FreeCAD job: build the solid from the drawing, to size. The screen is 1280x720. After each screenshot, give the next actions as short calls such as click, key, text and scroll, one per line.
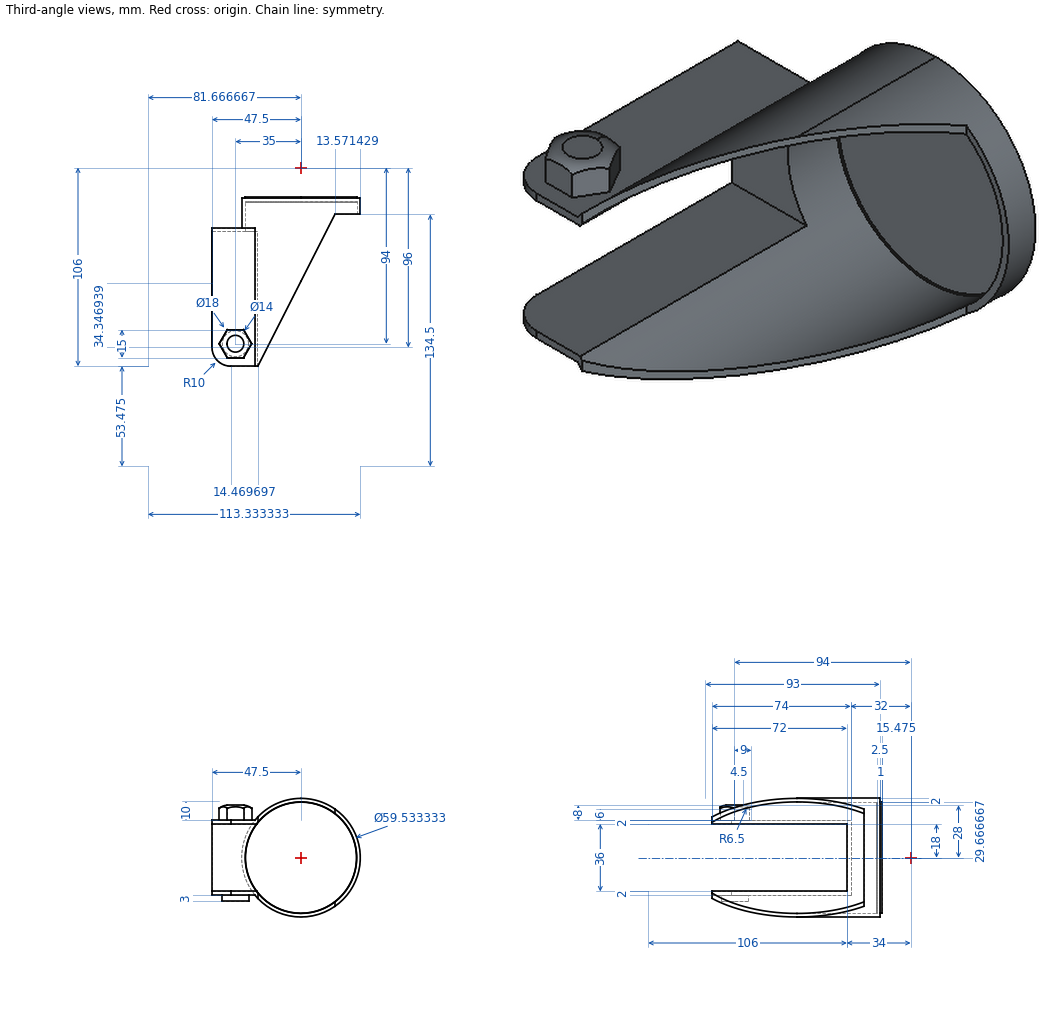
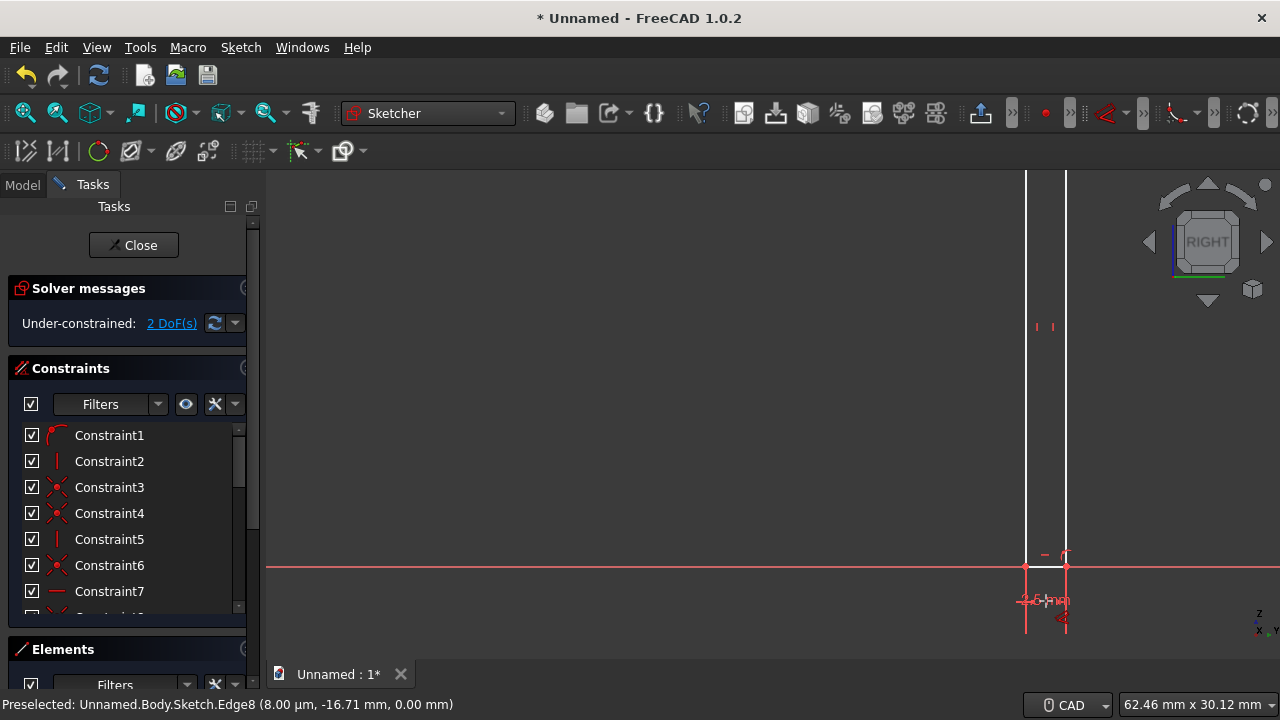
scroll(823, 460, down, 6)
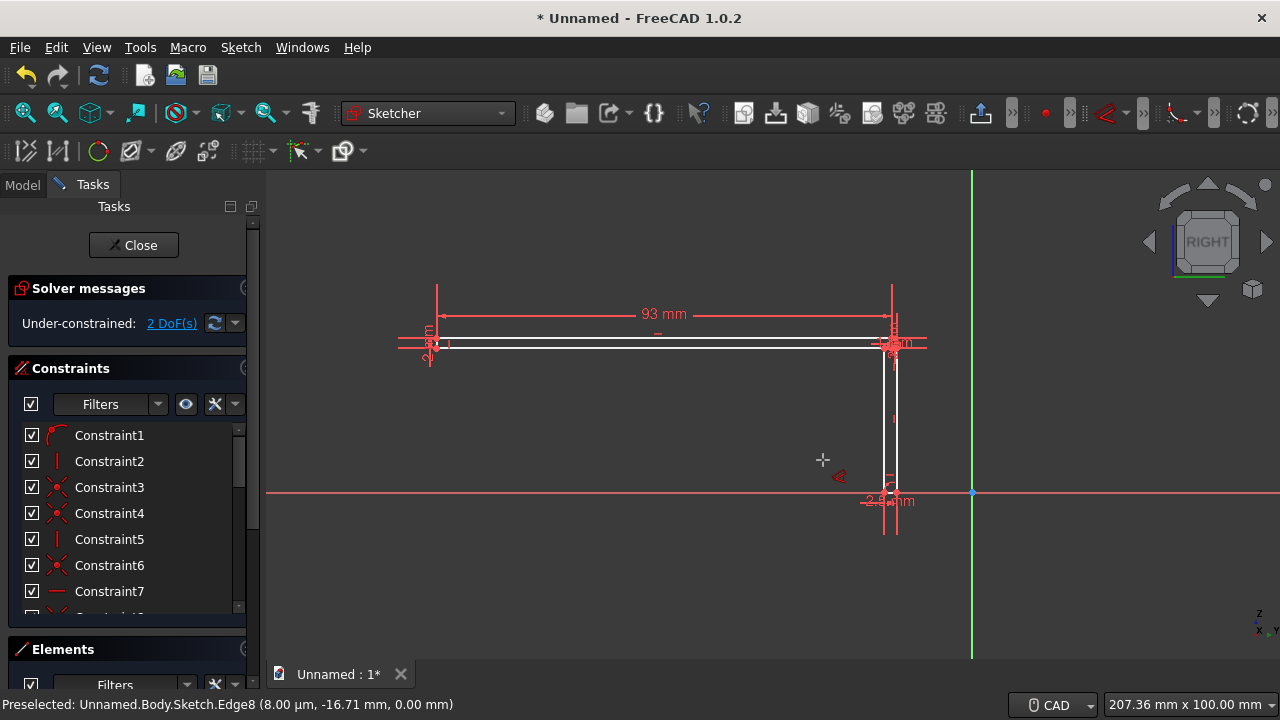
click(897, 493)
click(934, 527)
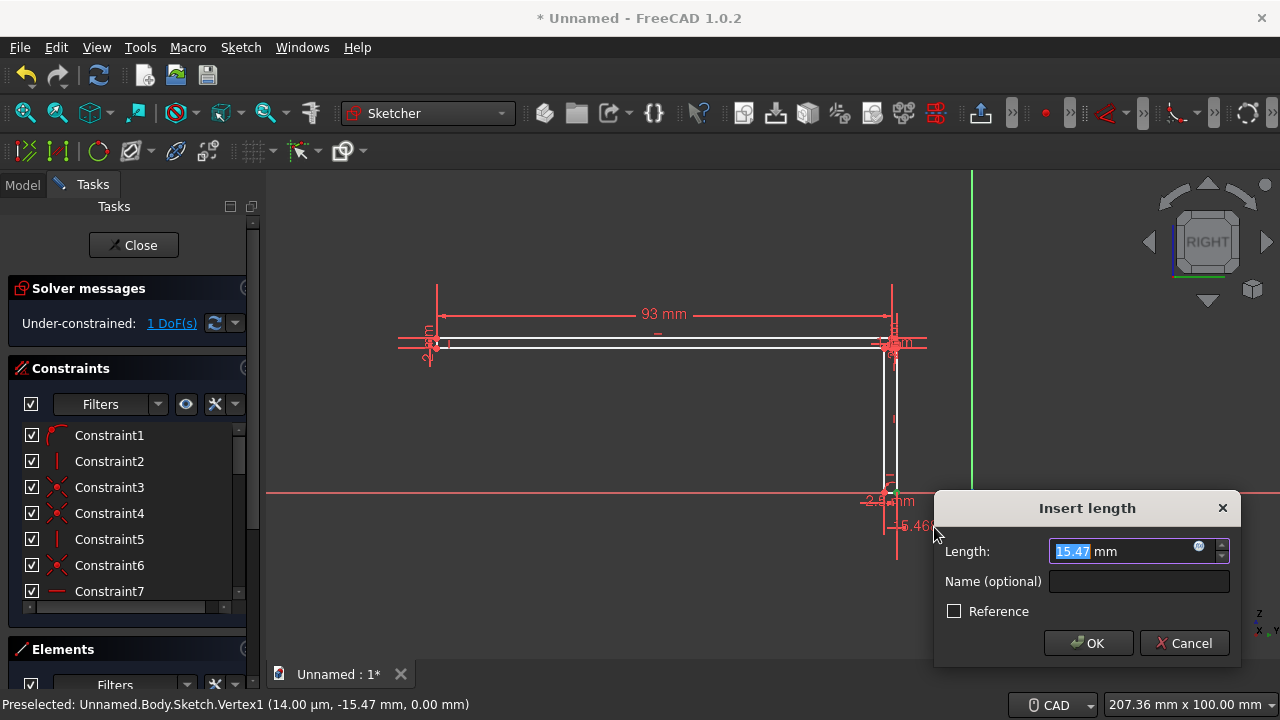
text(15.475)
key(Return)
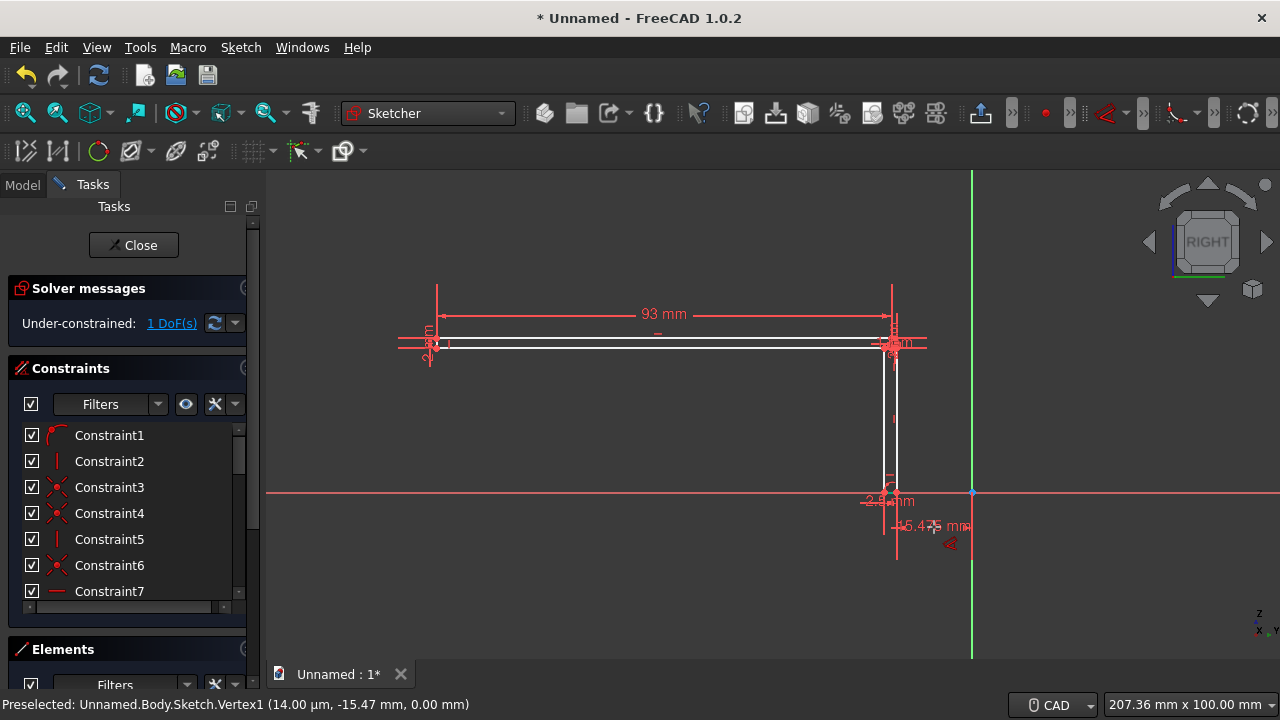
click(897, 449)
click(931, 420)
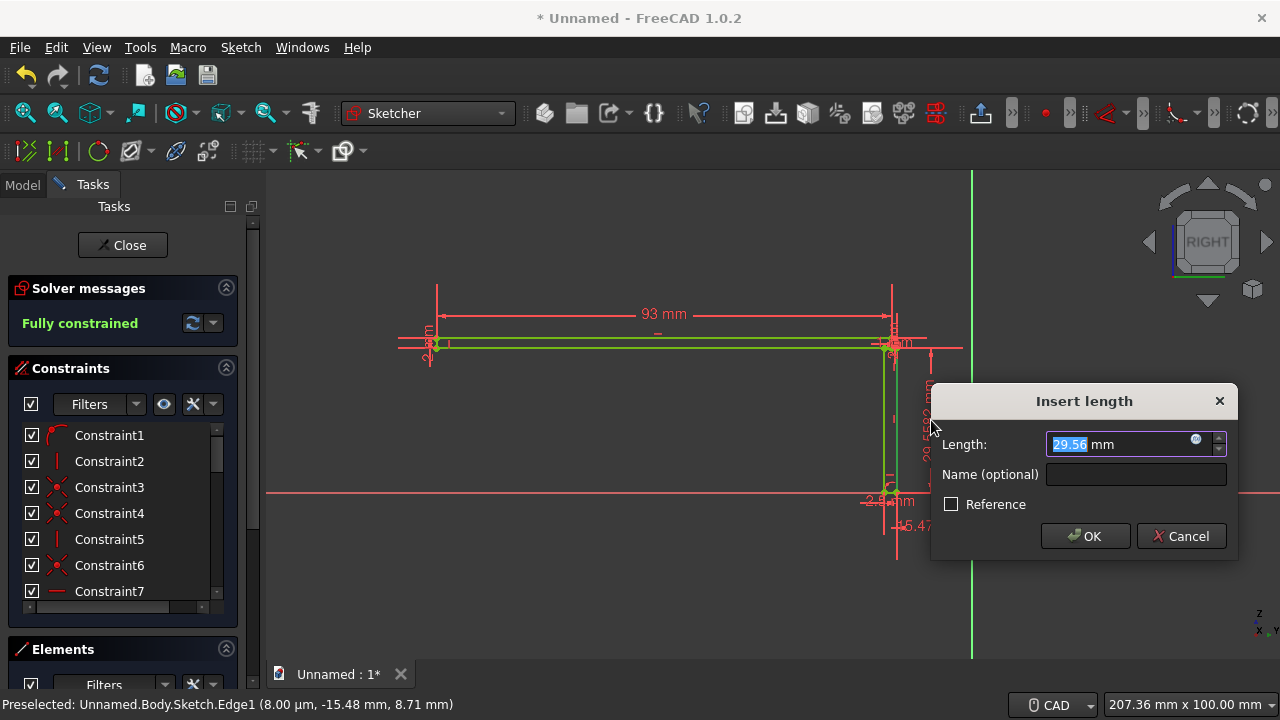
text(29.666667)
key(Return)
key(Escape)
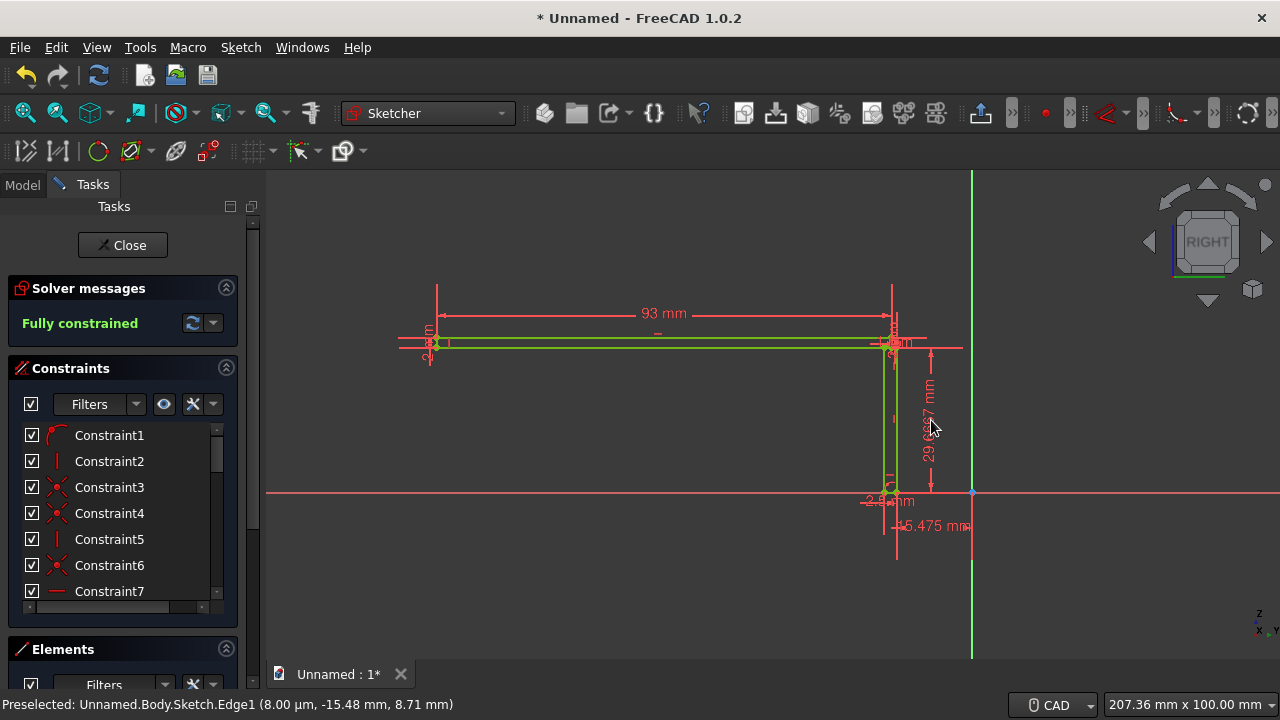
click(123, 245)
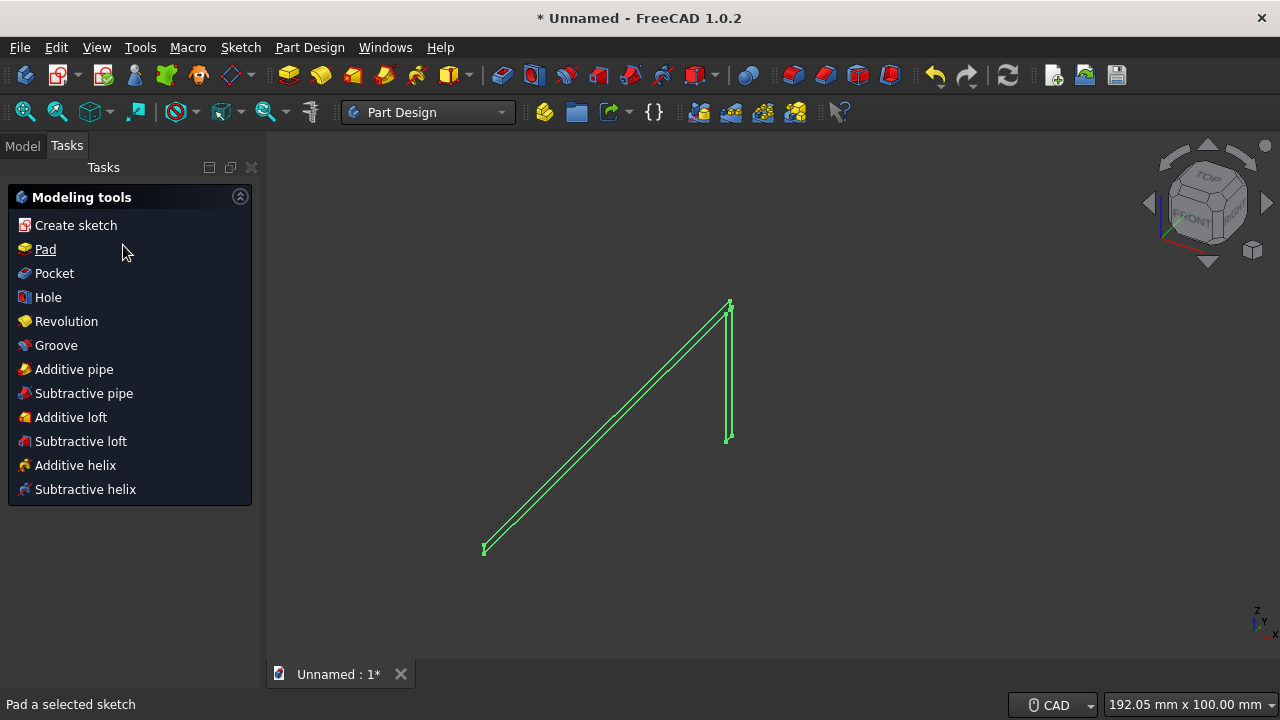
click(322, 76)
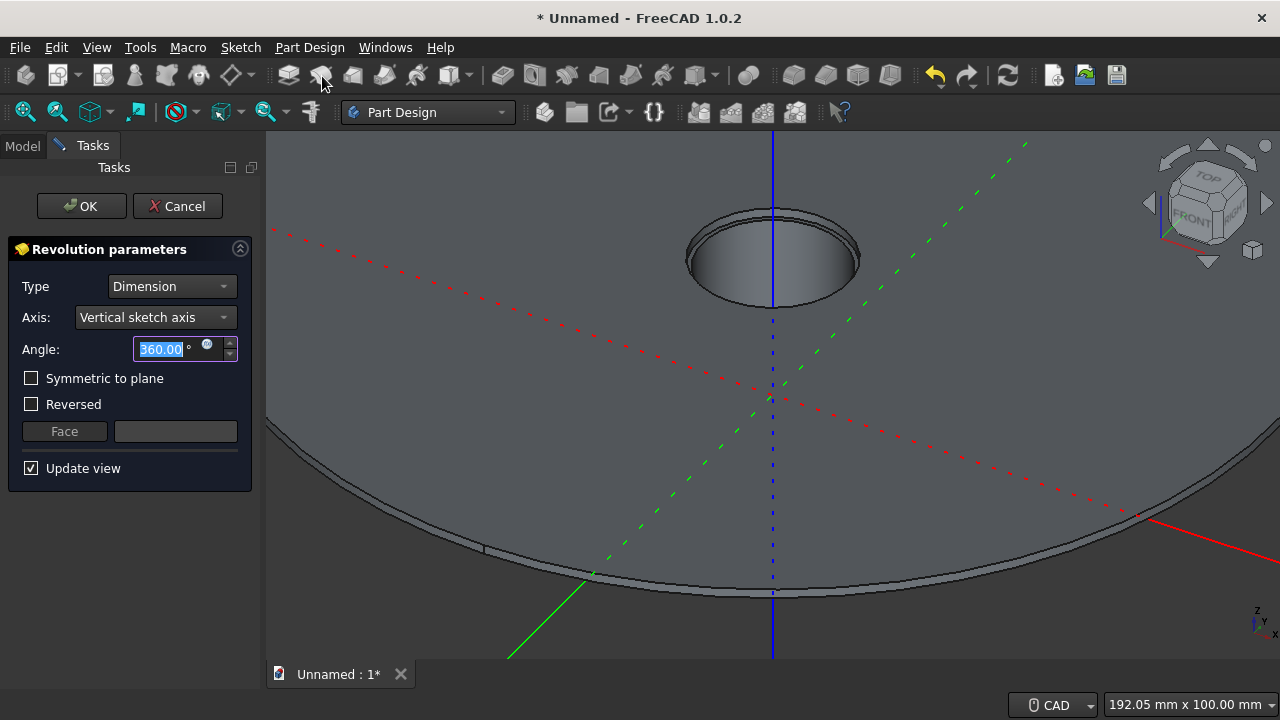
click(156, 318)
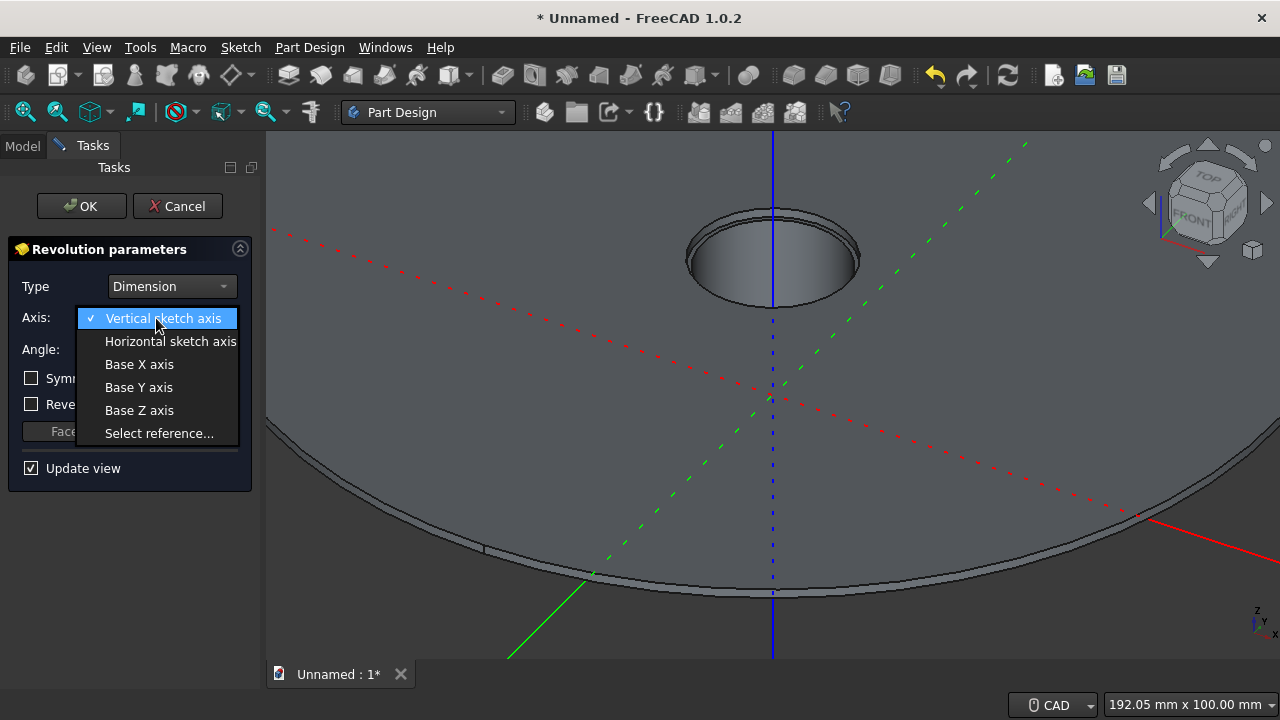
click(156, 342)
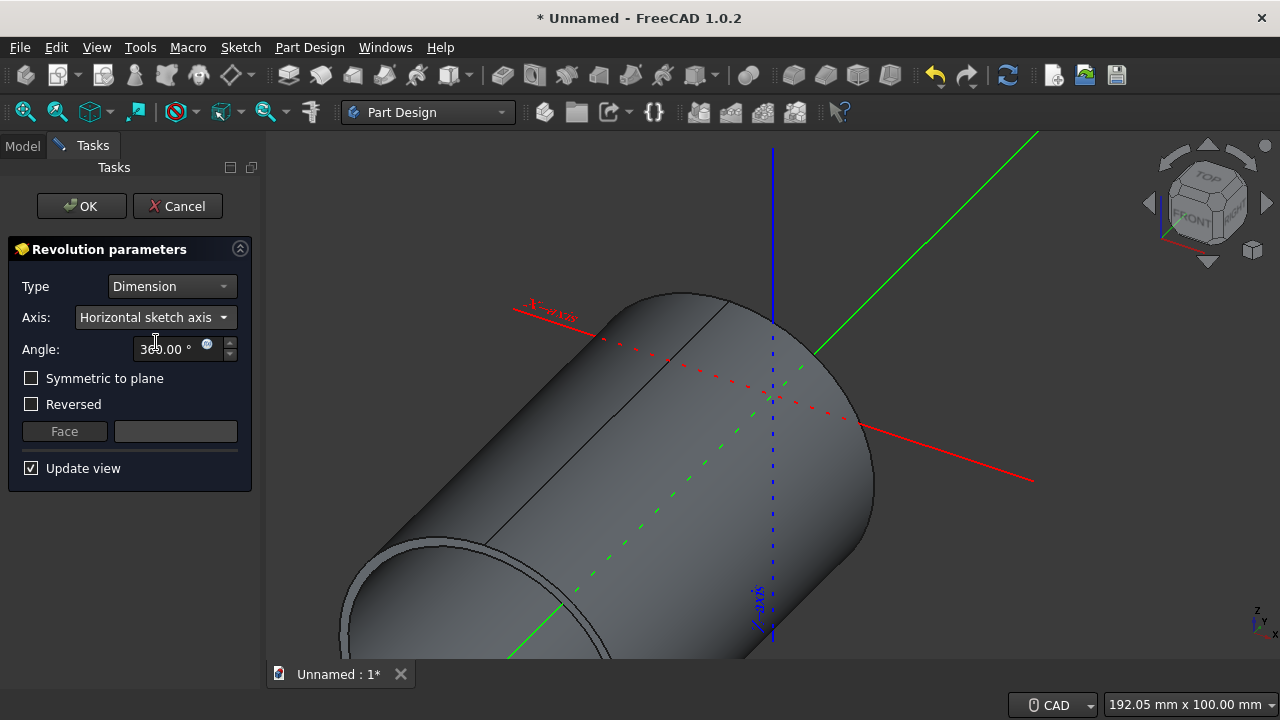
click(82, 206)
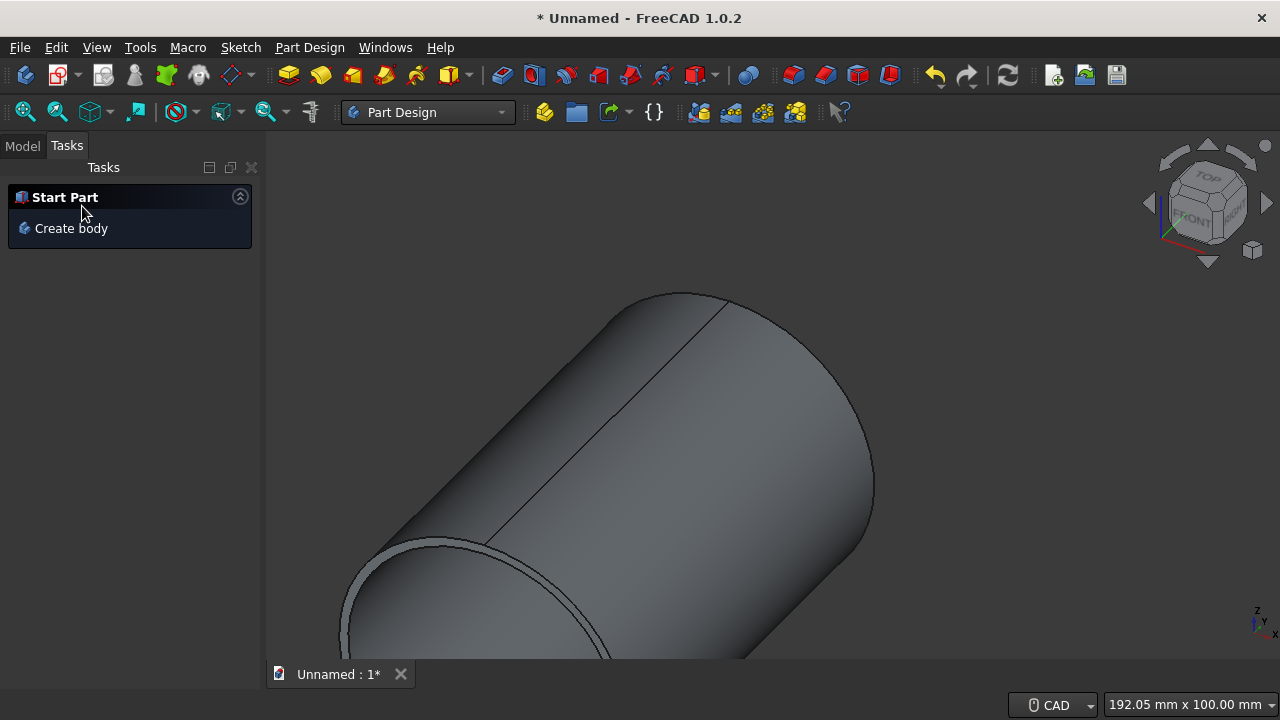
click(26, 112)